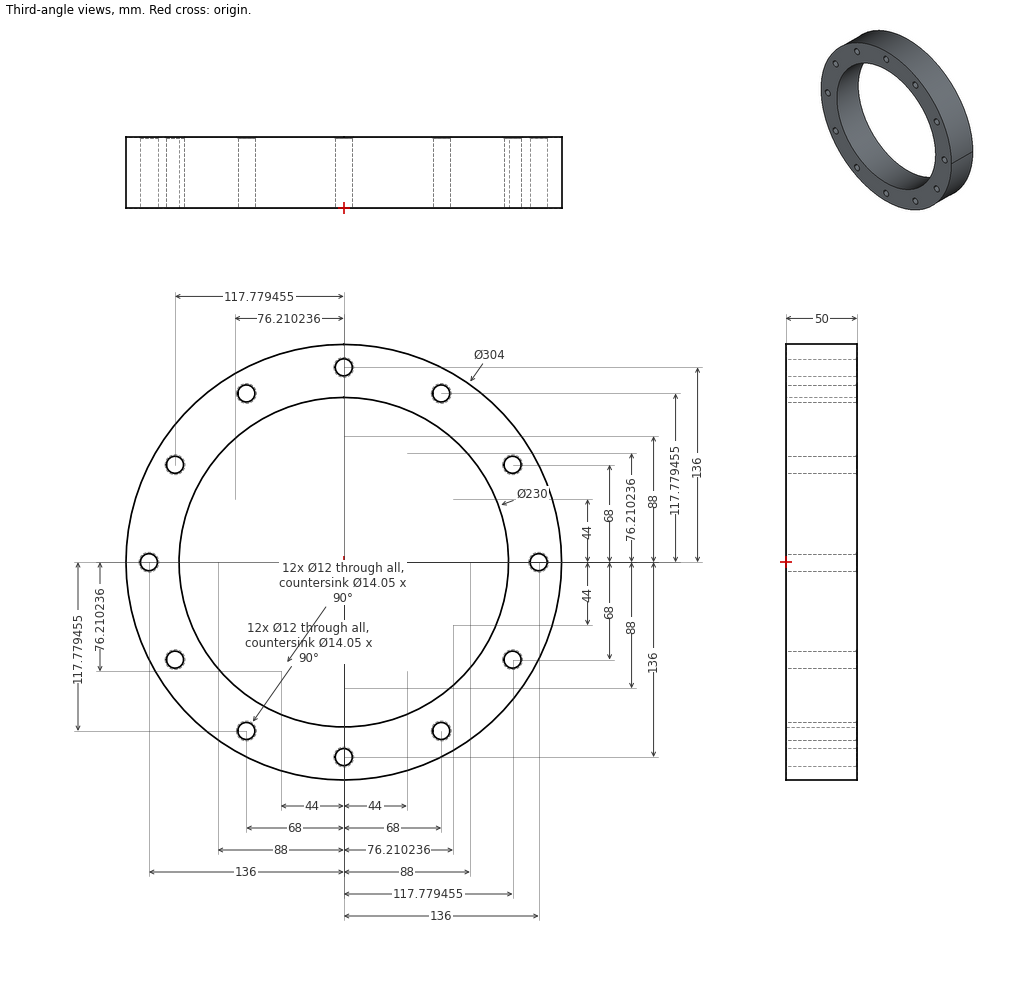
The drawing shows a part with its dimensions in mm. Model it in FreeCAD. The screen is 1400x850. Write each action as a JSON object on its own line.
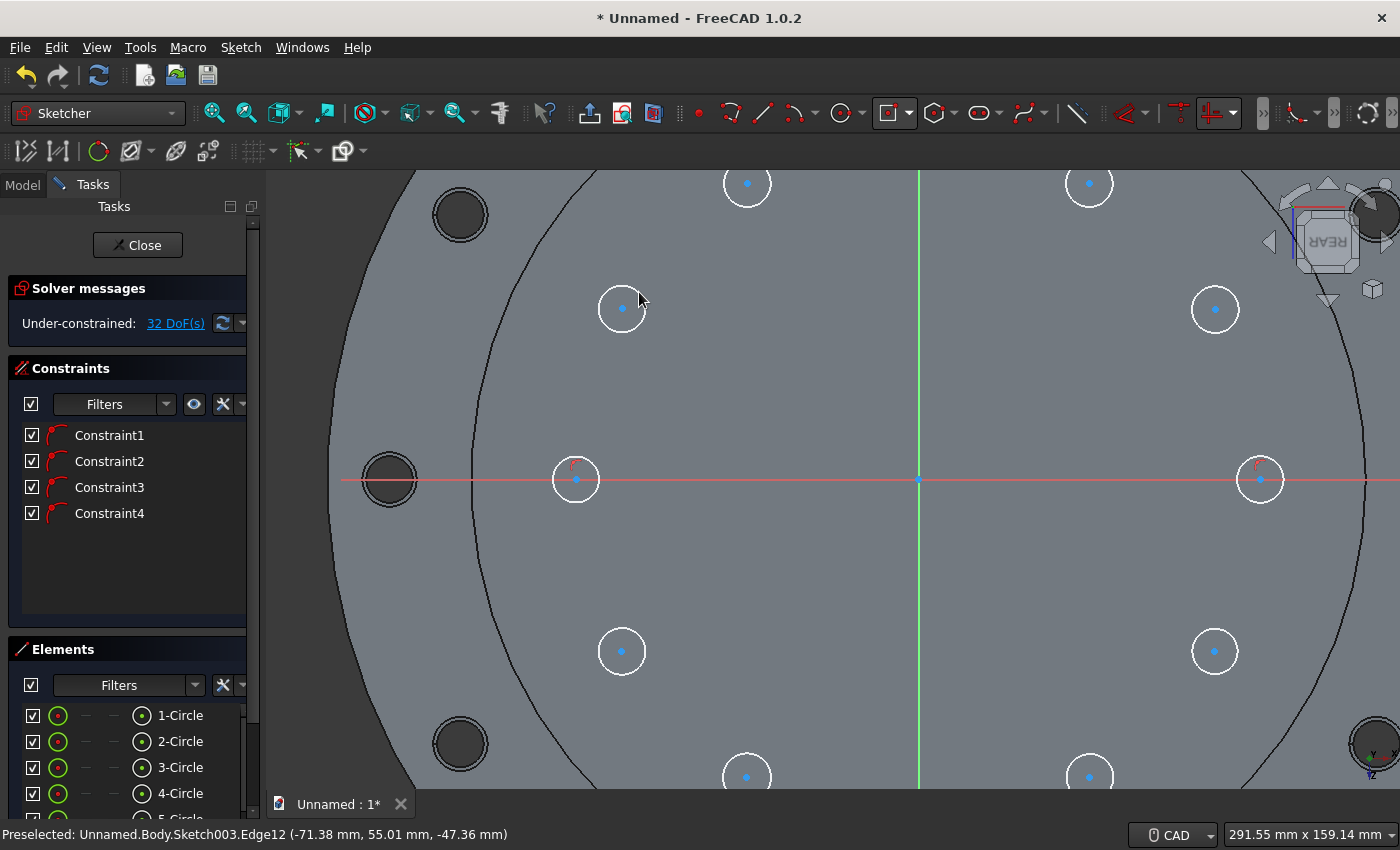
{"action": "left_click", "coordinate": [731, 200]}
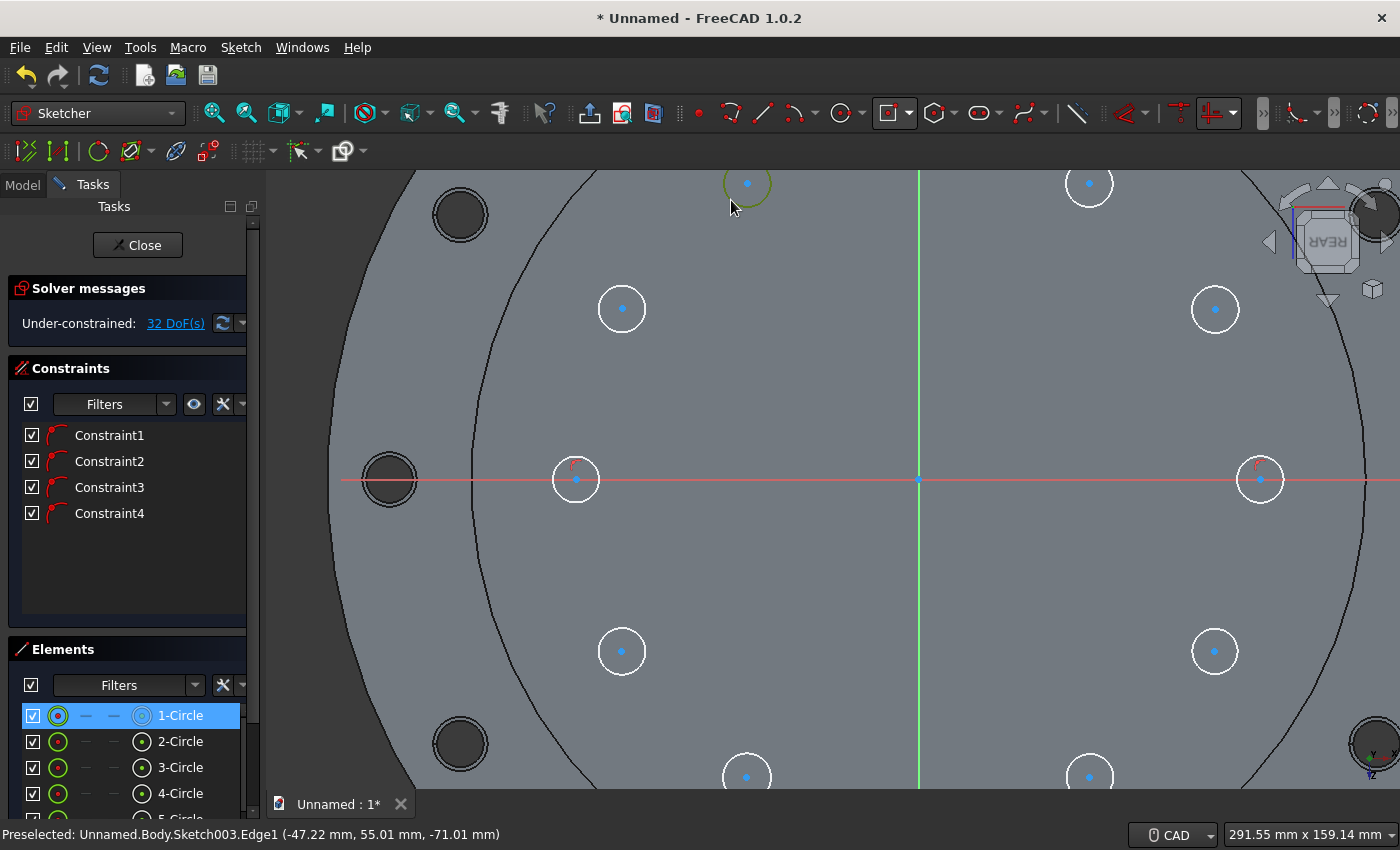
{"action": "scroll", "coordinate": [577, 480], "scroll_direction": "down", "scroll_amount": 3}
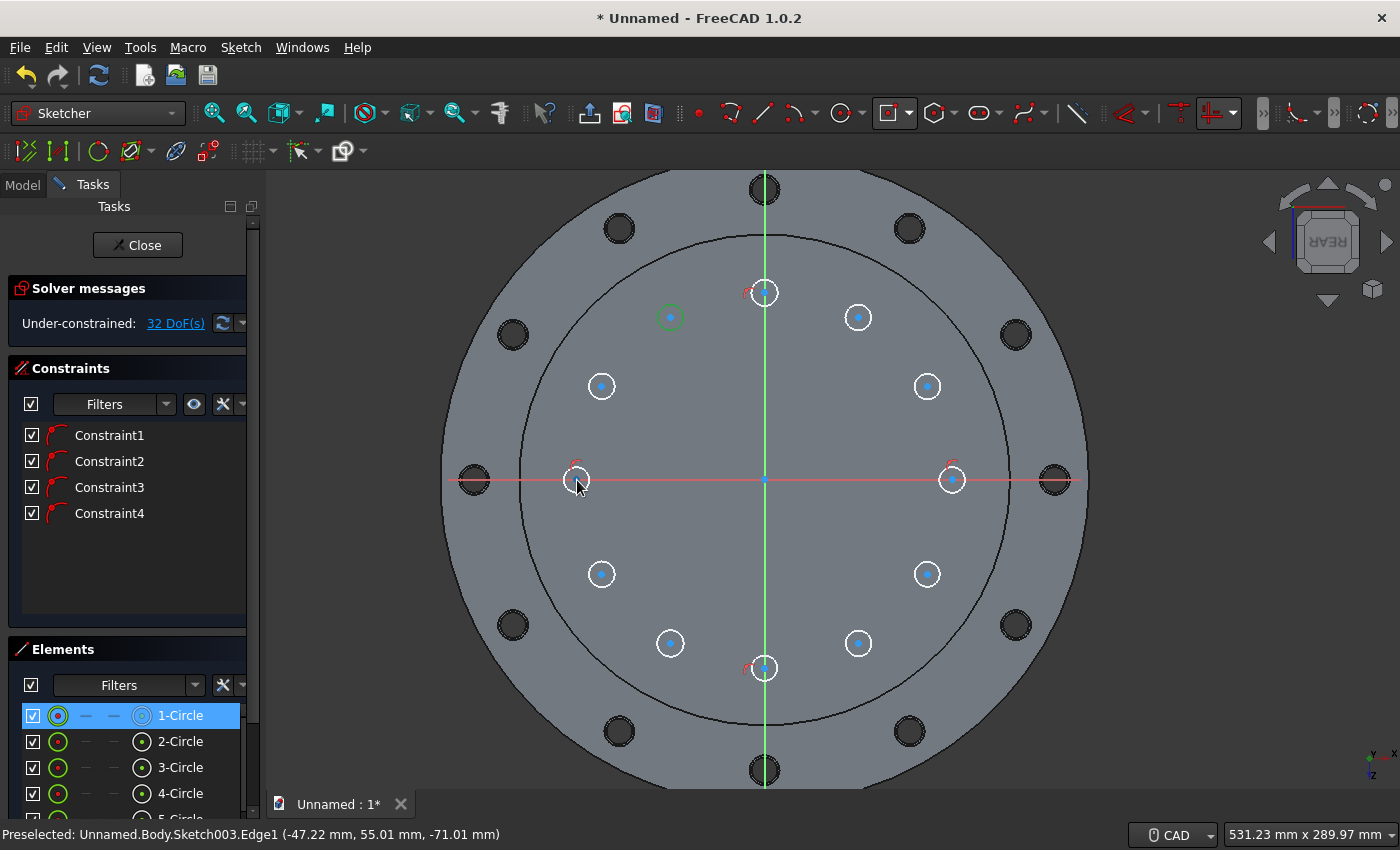
{"action": "scroll", "coordinate": [774, 284], "scroll_direction": "up", "scroll_amount": 3}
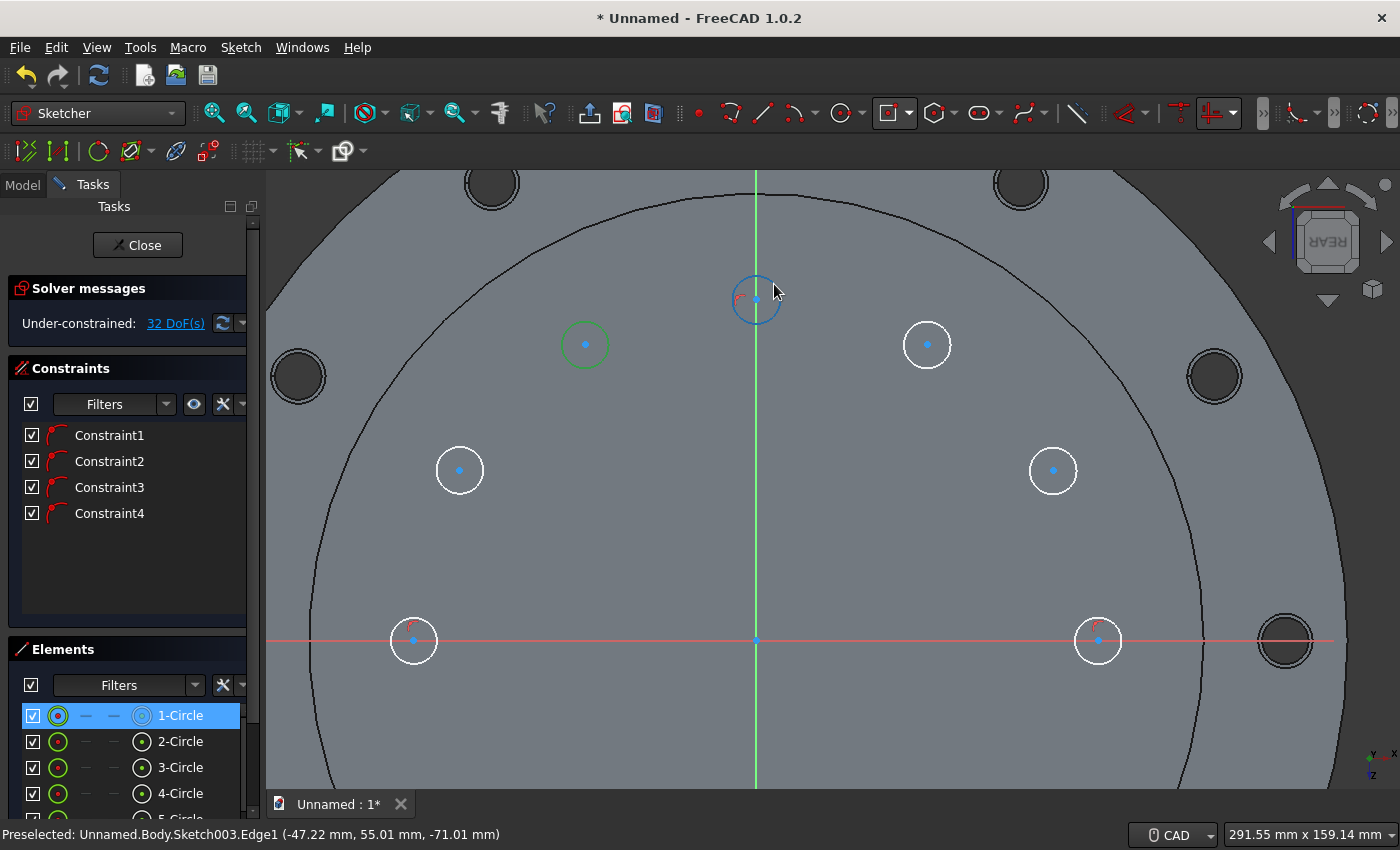
{"action": "left_click", "coordinate": [773, 283]}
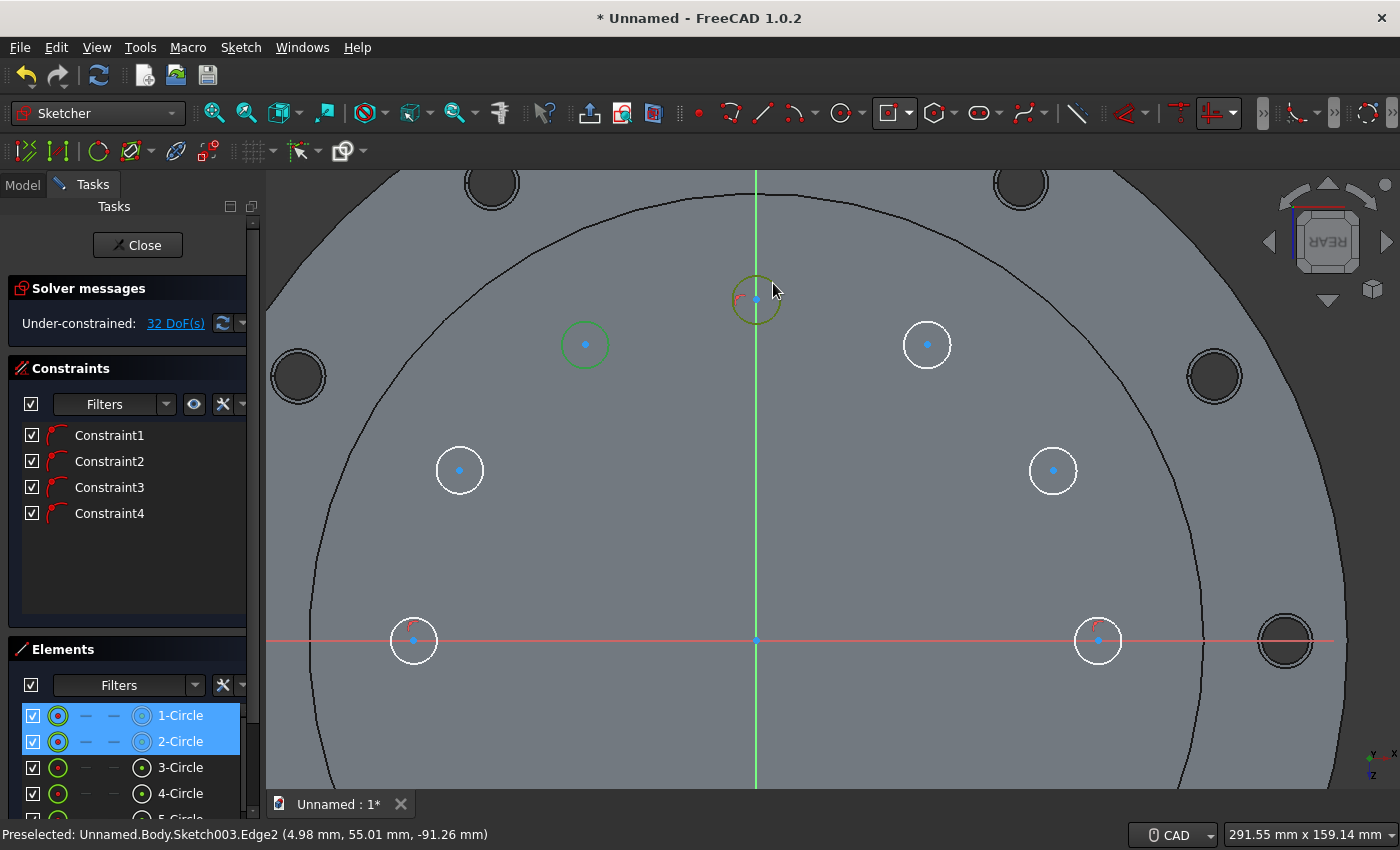
{"action": "left_click", "coordinate": [944, 328]}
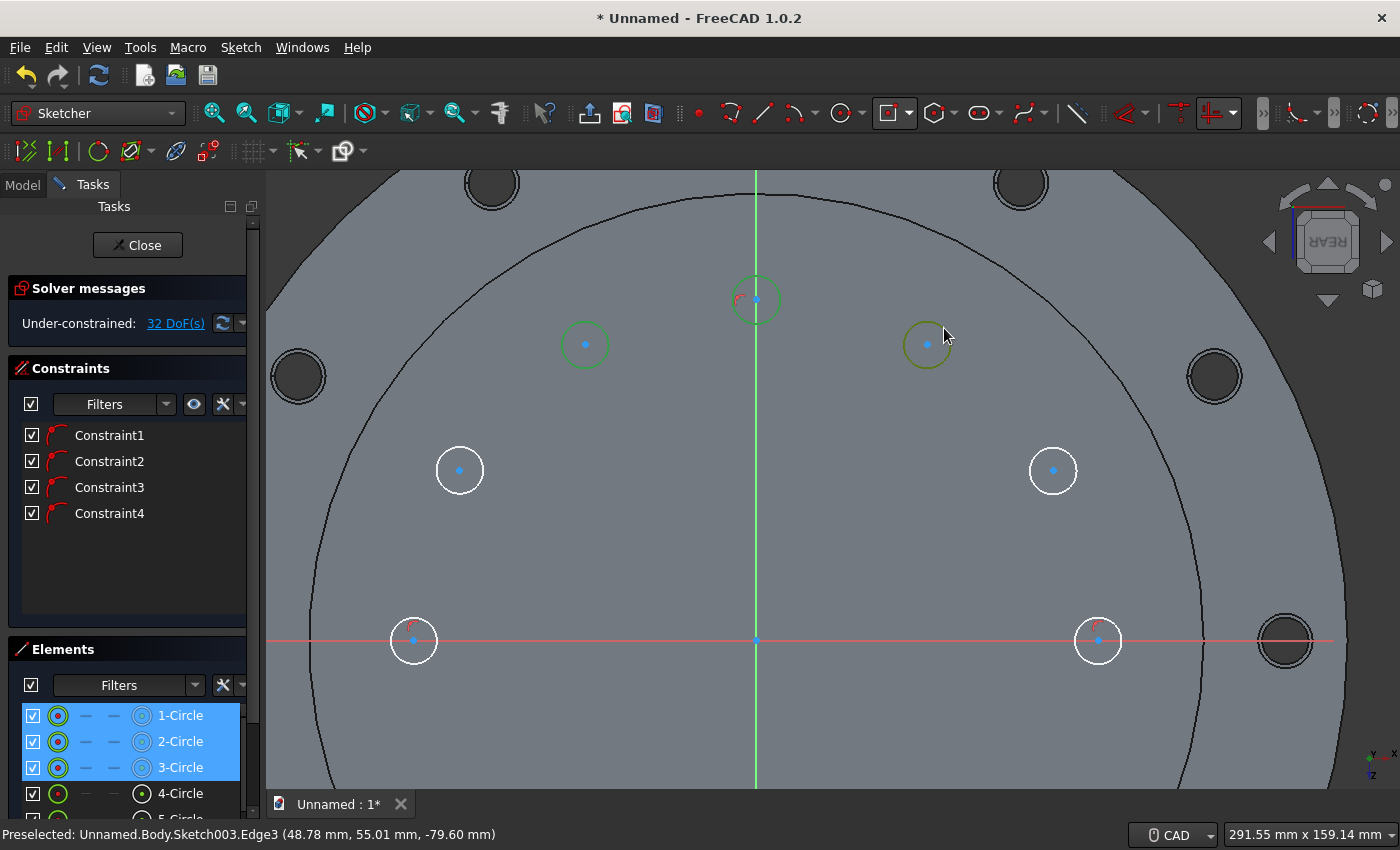
{"action": "left_click", "coordinate": [1070, 454]}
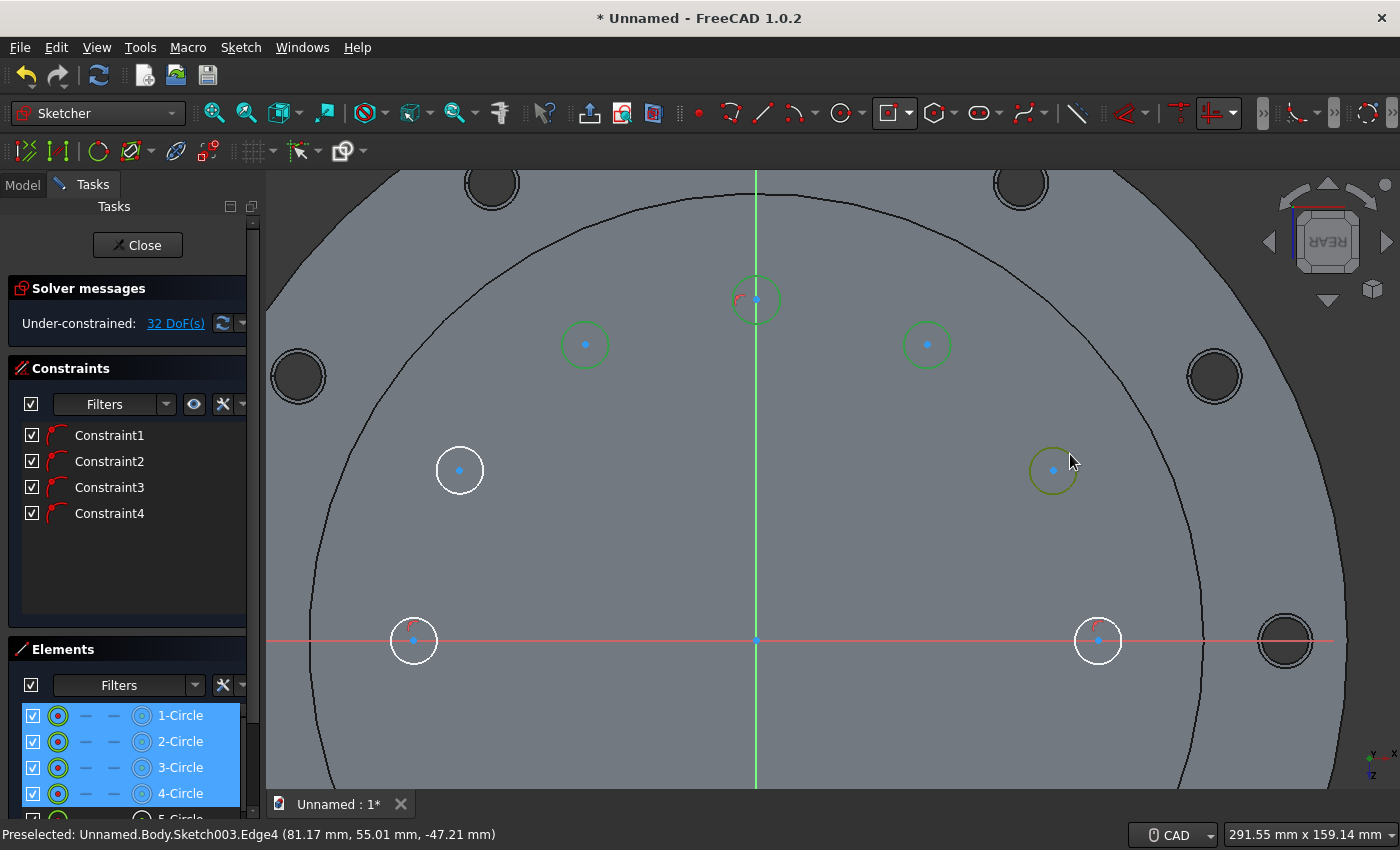
{"action": "left_click", "coordinate": [1115, 624]}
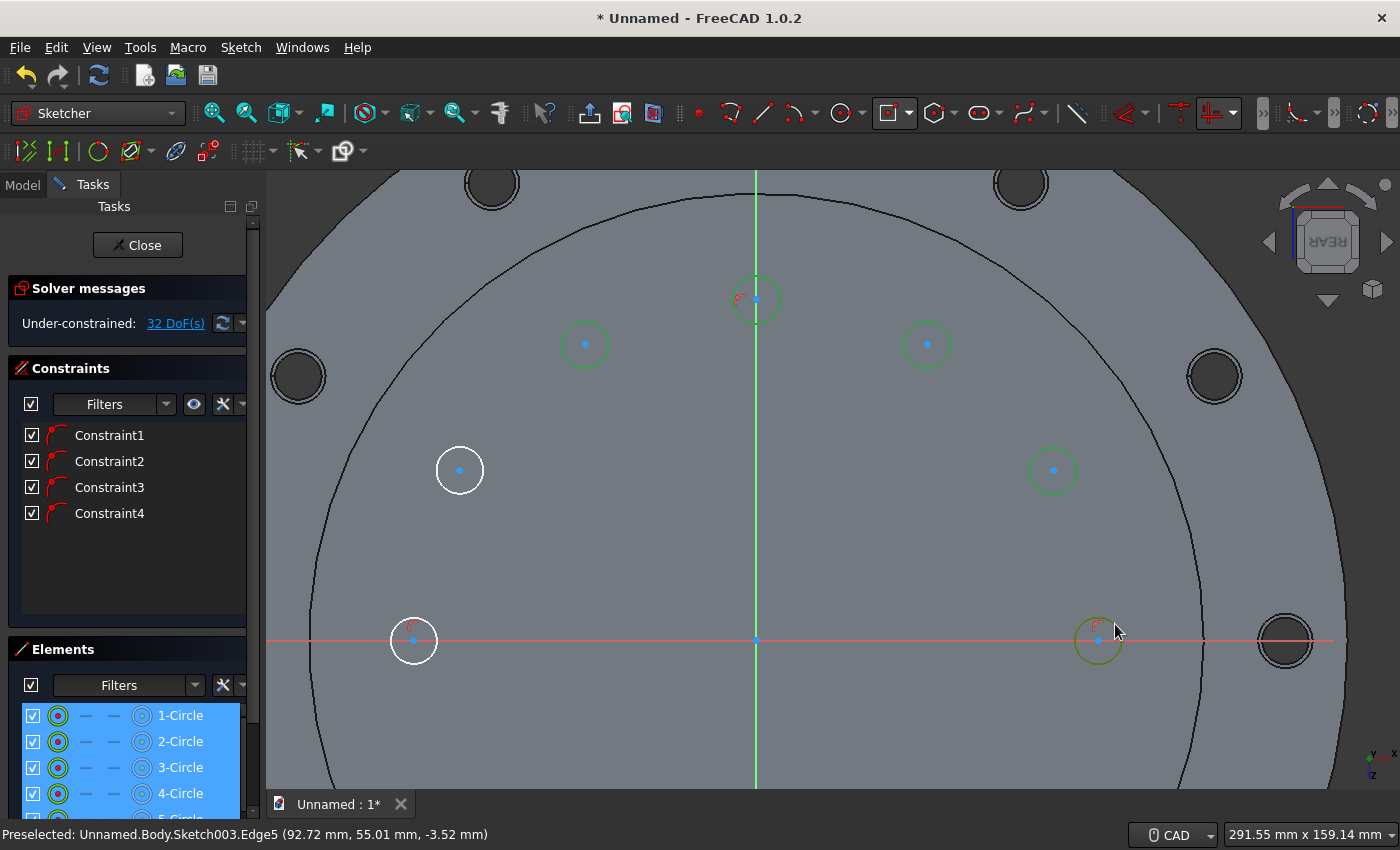
{"action": "scroll", "coordinate": [774, 283], "scroll_direction": "down", "scroll_amount": 3}